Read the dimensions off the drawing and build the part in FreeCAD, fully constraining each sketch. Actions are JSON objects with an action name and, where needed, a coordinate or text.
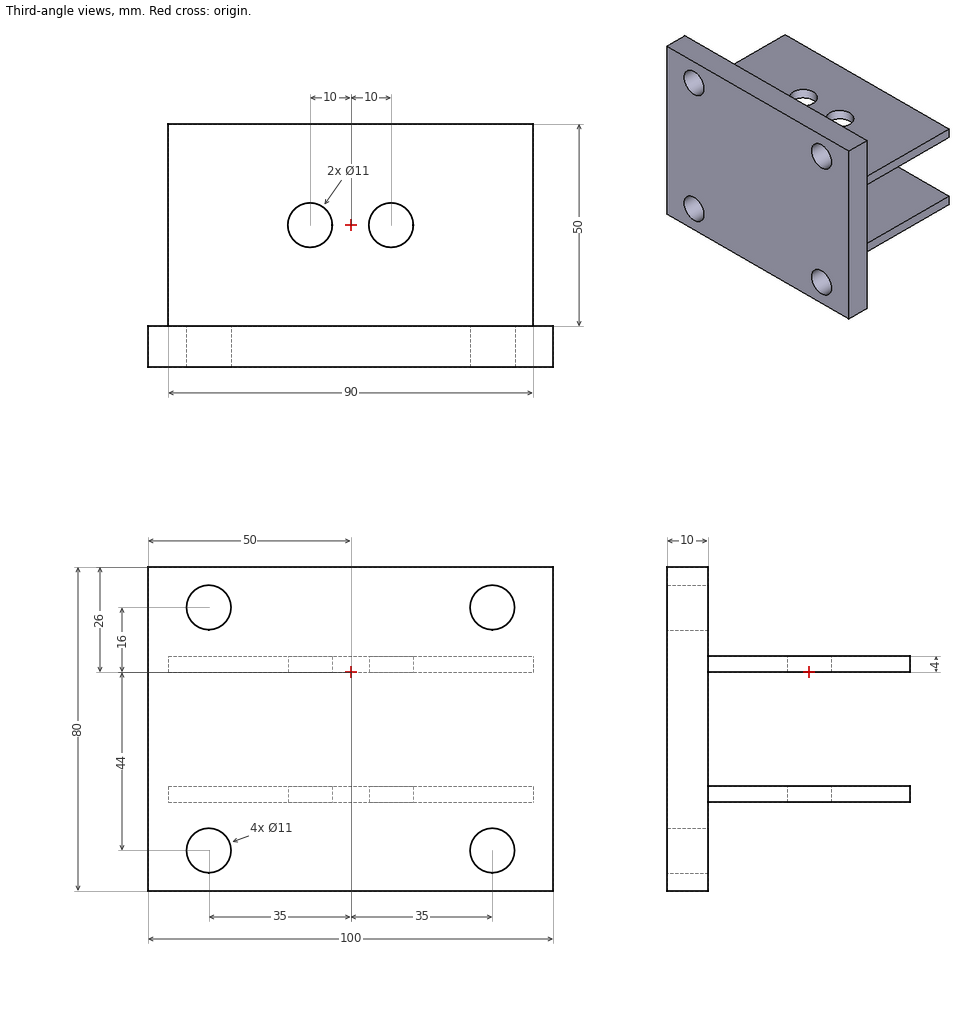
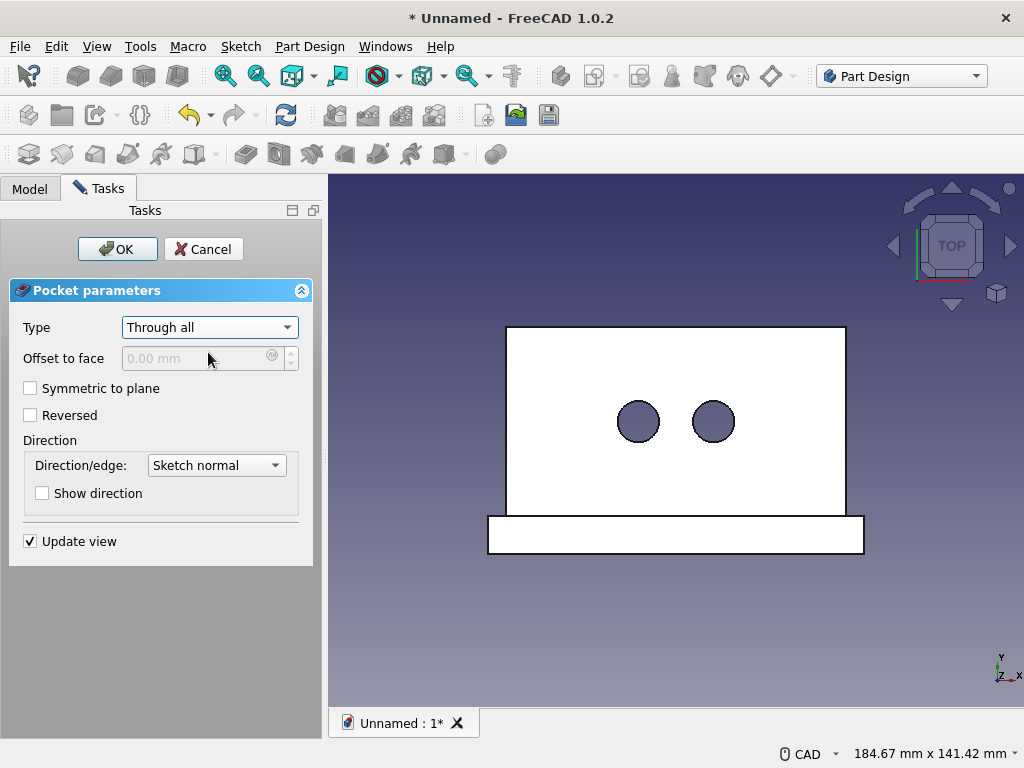
{"action": "left_click", "coordinate": [118, 249]}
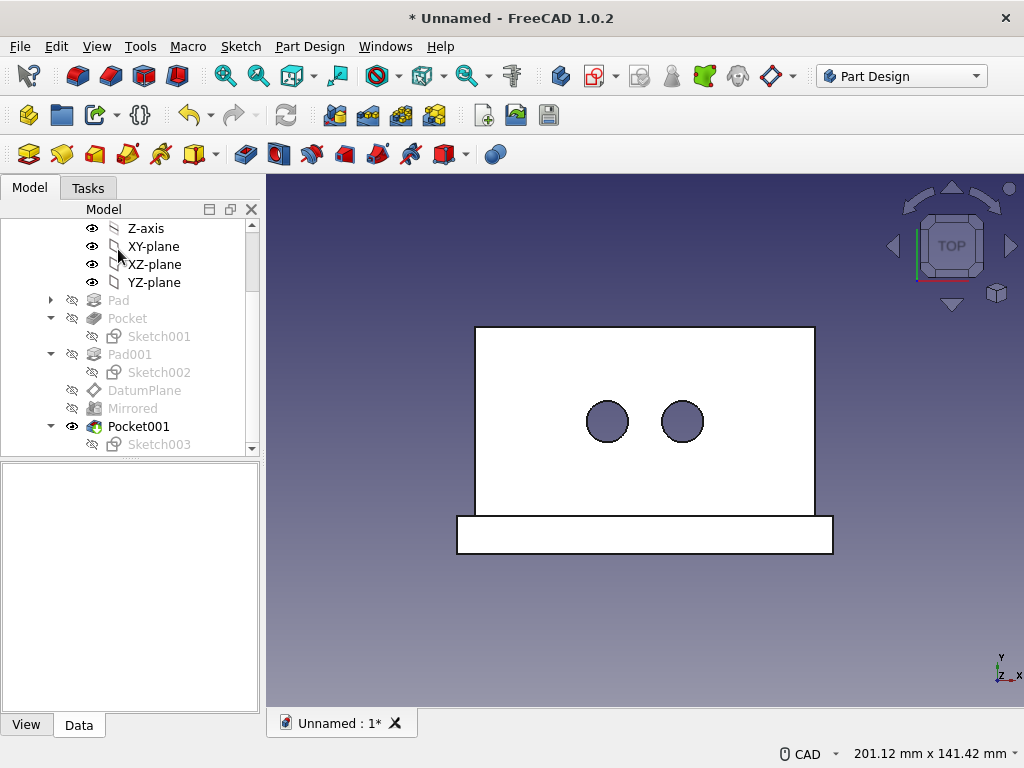
{"action": "key", "text": "0"}